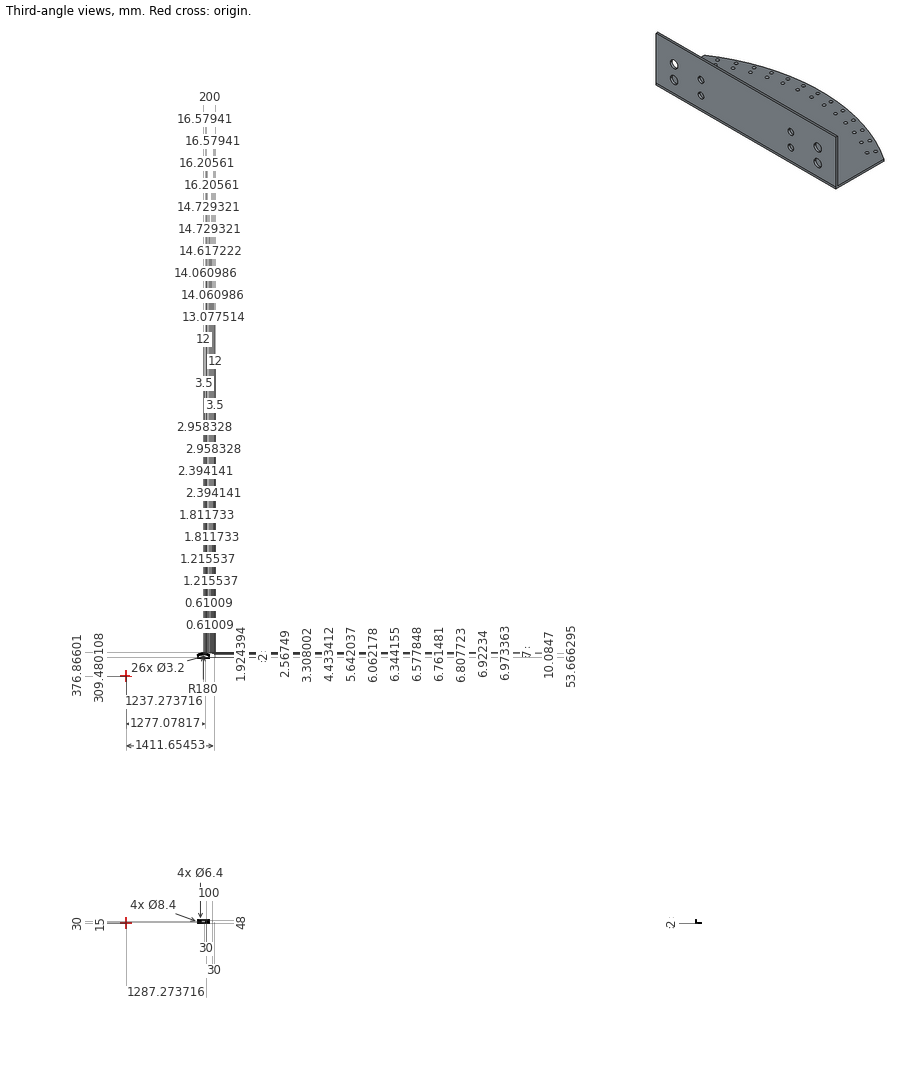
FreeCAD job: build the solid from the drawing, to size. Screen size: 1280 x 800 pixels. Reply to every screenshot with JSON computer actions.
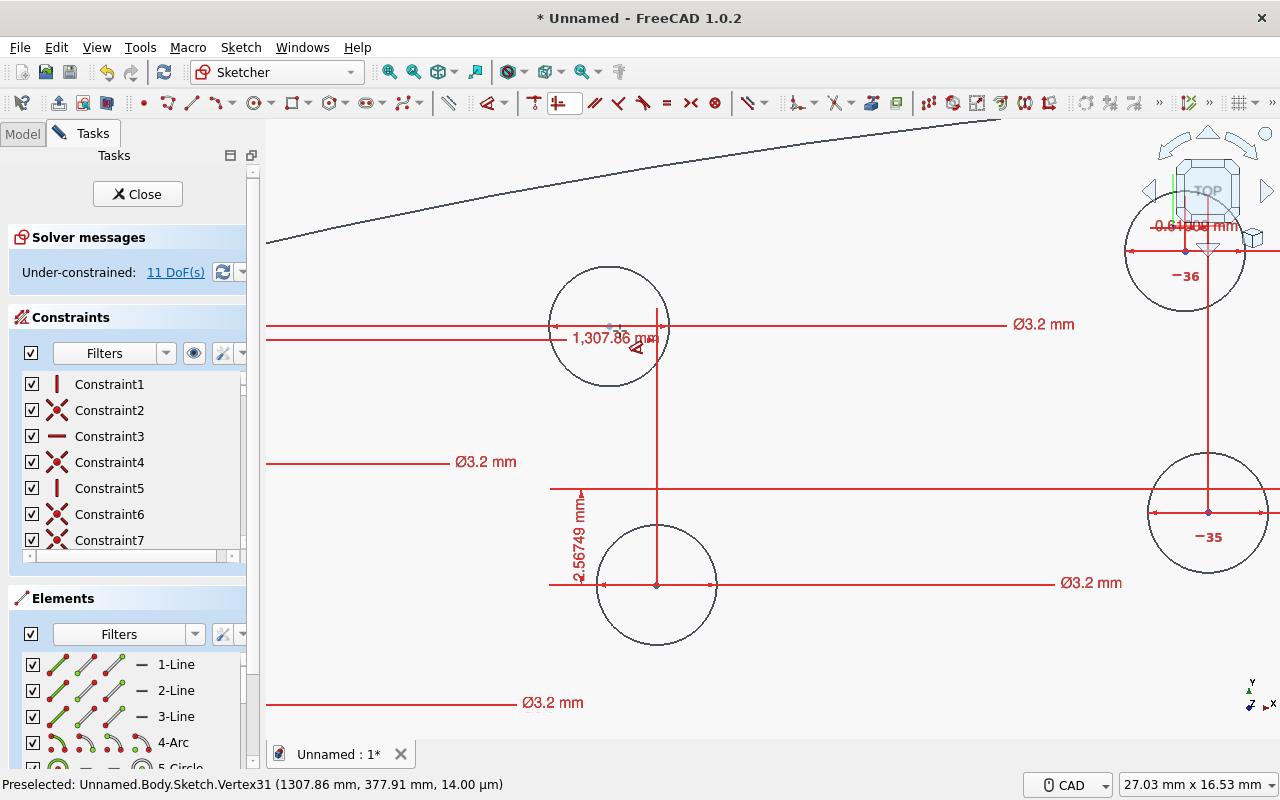
{"action": "left_click", "coordinate": [609, 326]}
{"action": "left_click", "coordinate": [633, 292]}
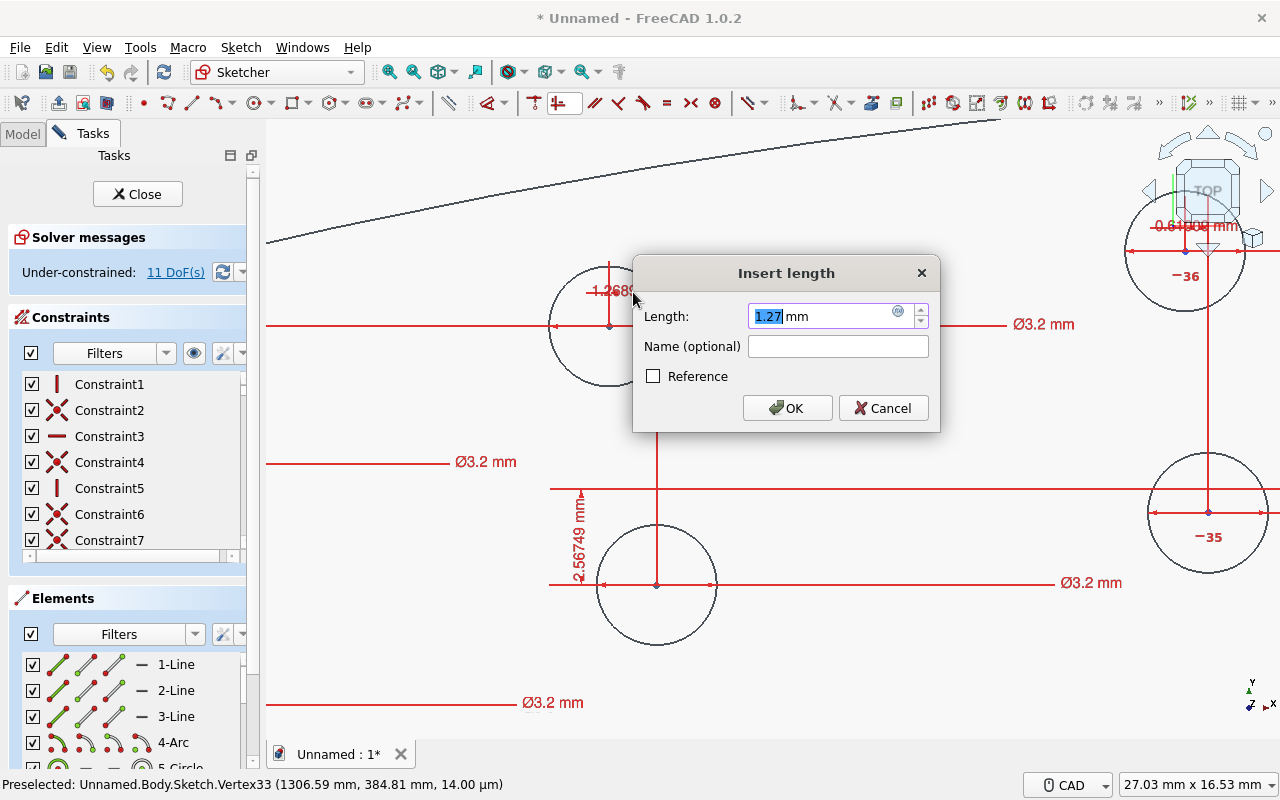
{"action": "type", "text": "1.215537"}
{"action": "key", "text": "Return"}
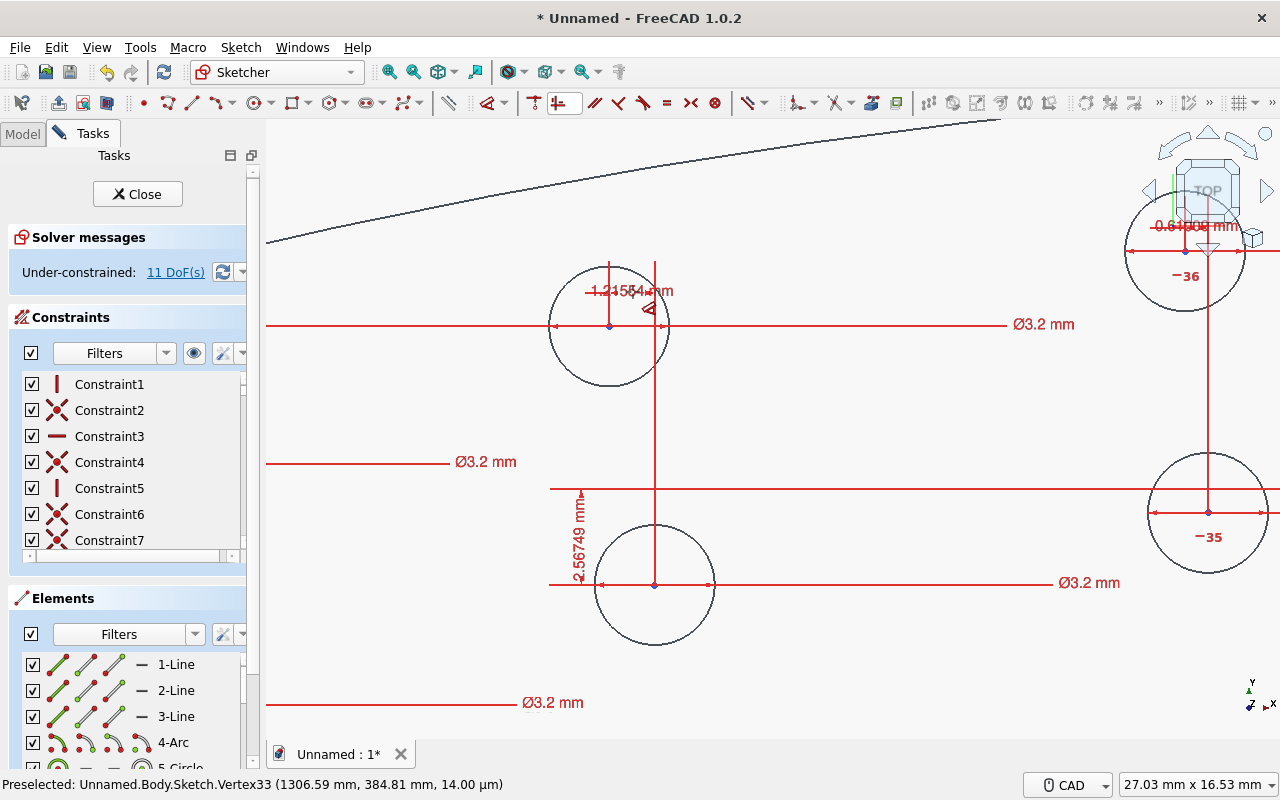
{"action": "scroll", "coordinate": [620, 331], "scroll_direction": "down", "scroll_amount": 13}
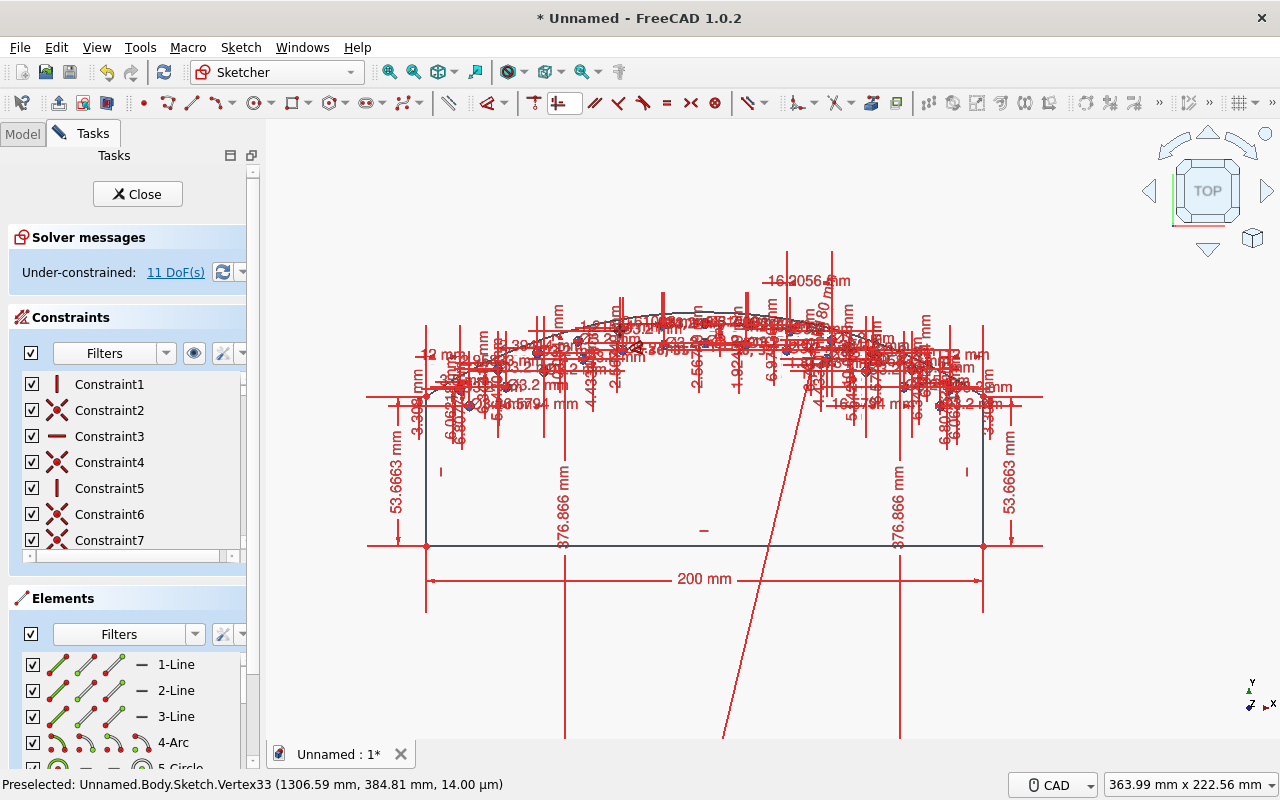
{"action": "scroll", "coordinate": [583, 359], "scroll_direction": "up", "scroll_amount": 11}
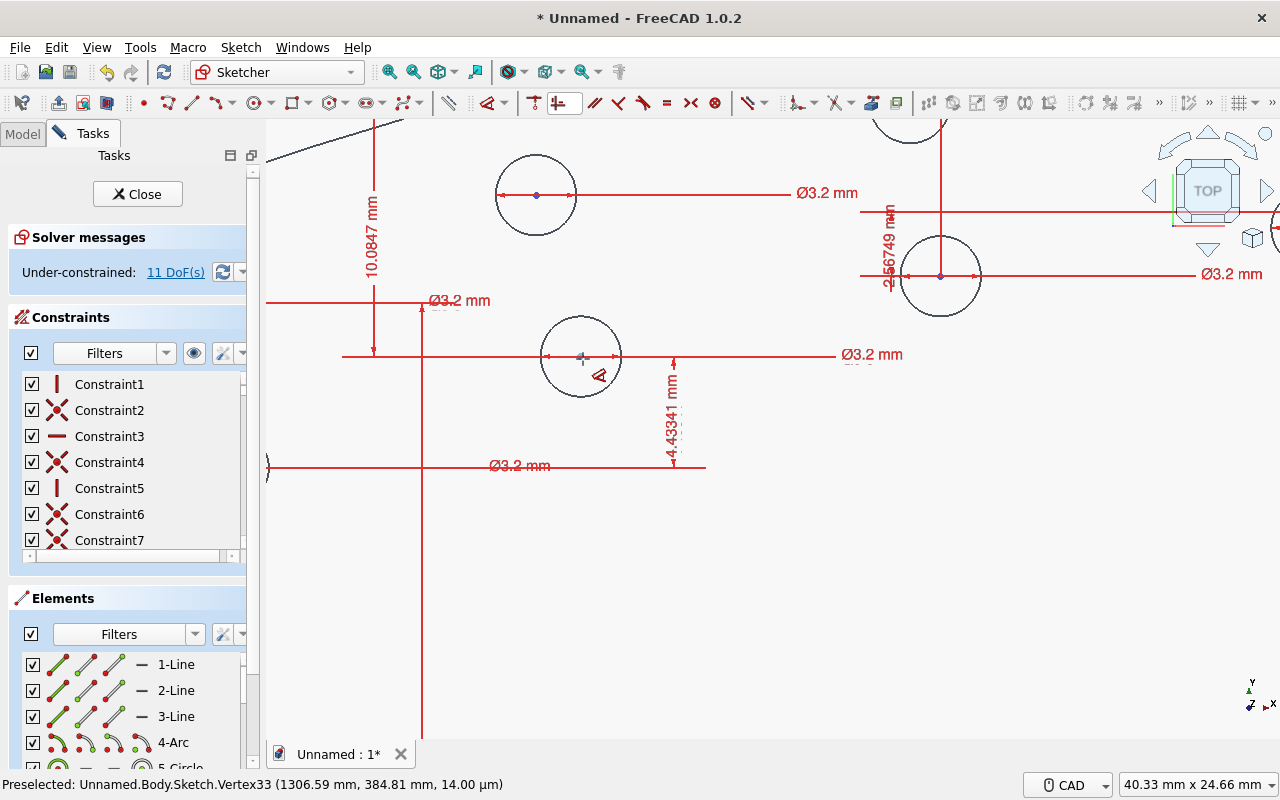
{"action": "left_click", "coordinate": [581, 357]}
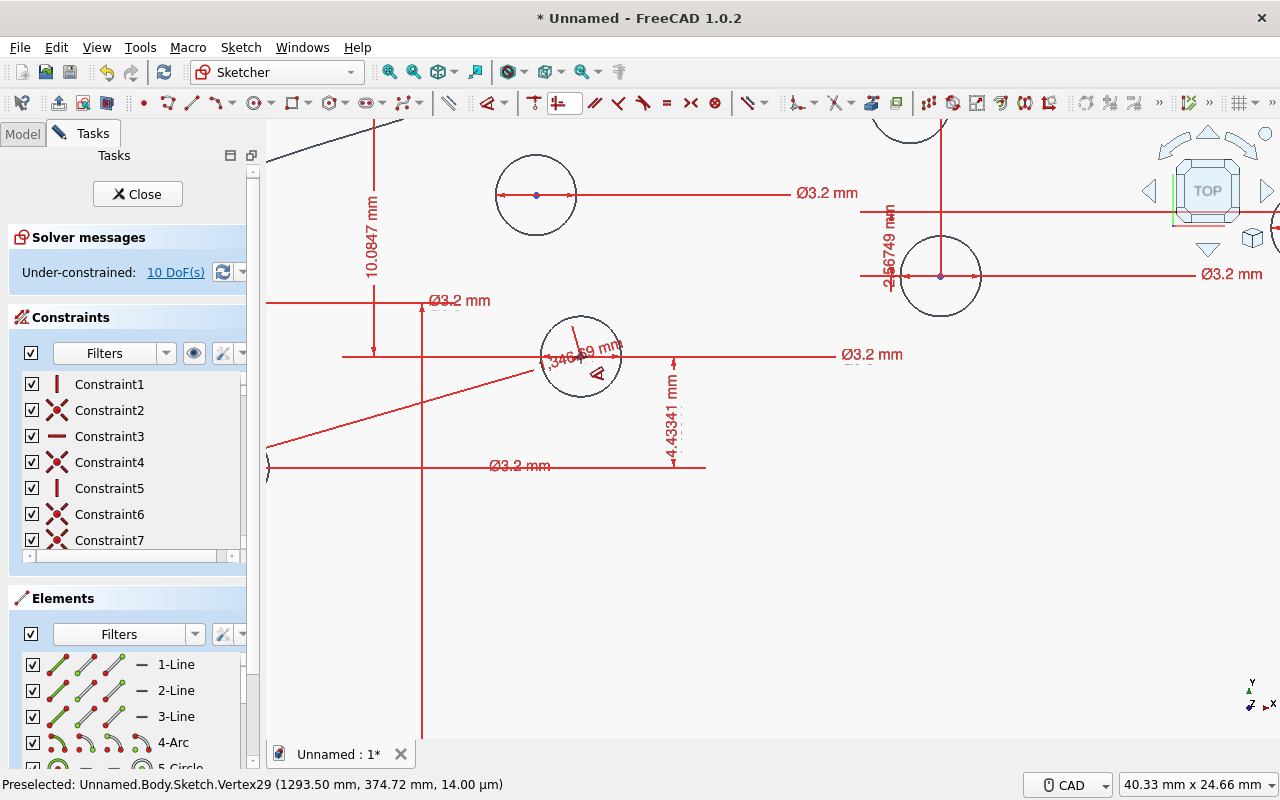
{"action": "left_click", "coordinate": [536, 195]}
{"action": "left_click", "coordinate": [559, 415]}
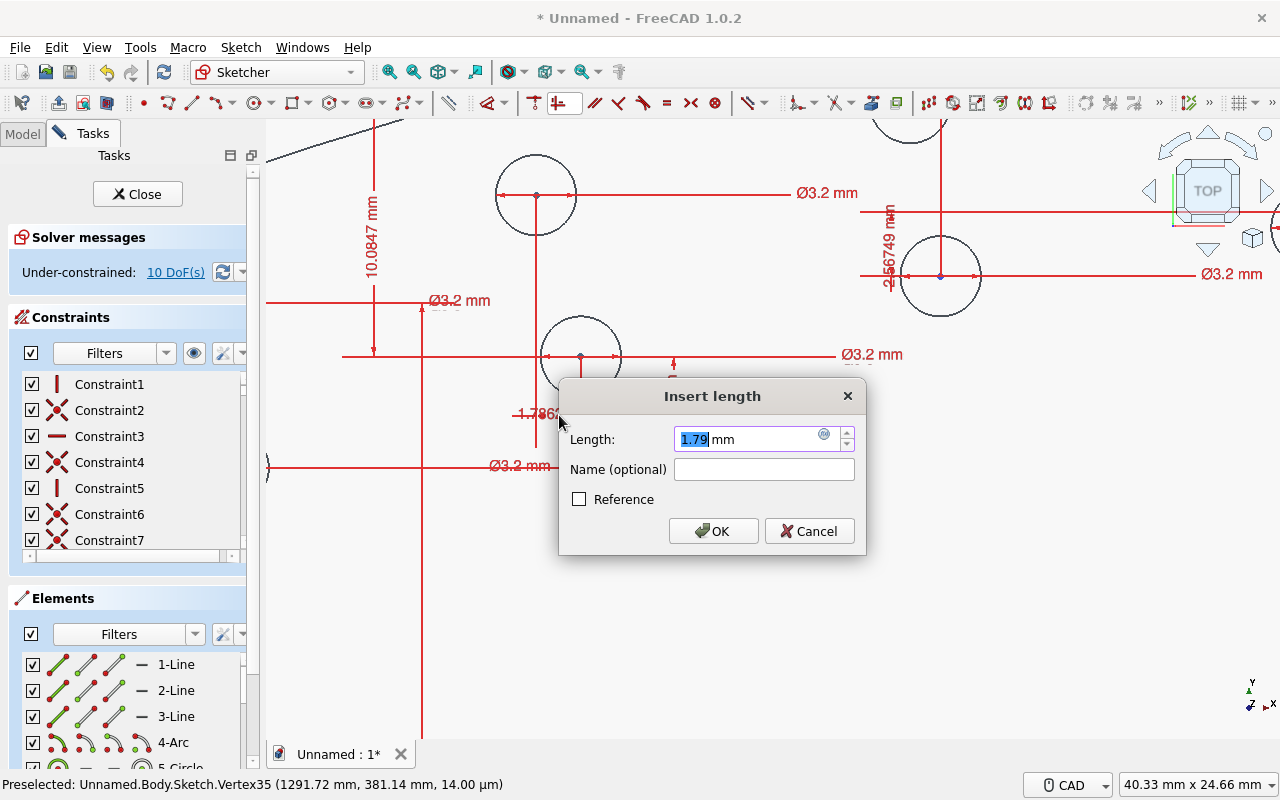
{"action": "type", "text": "1.811733"}
{"action": "key", "text": "Return"}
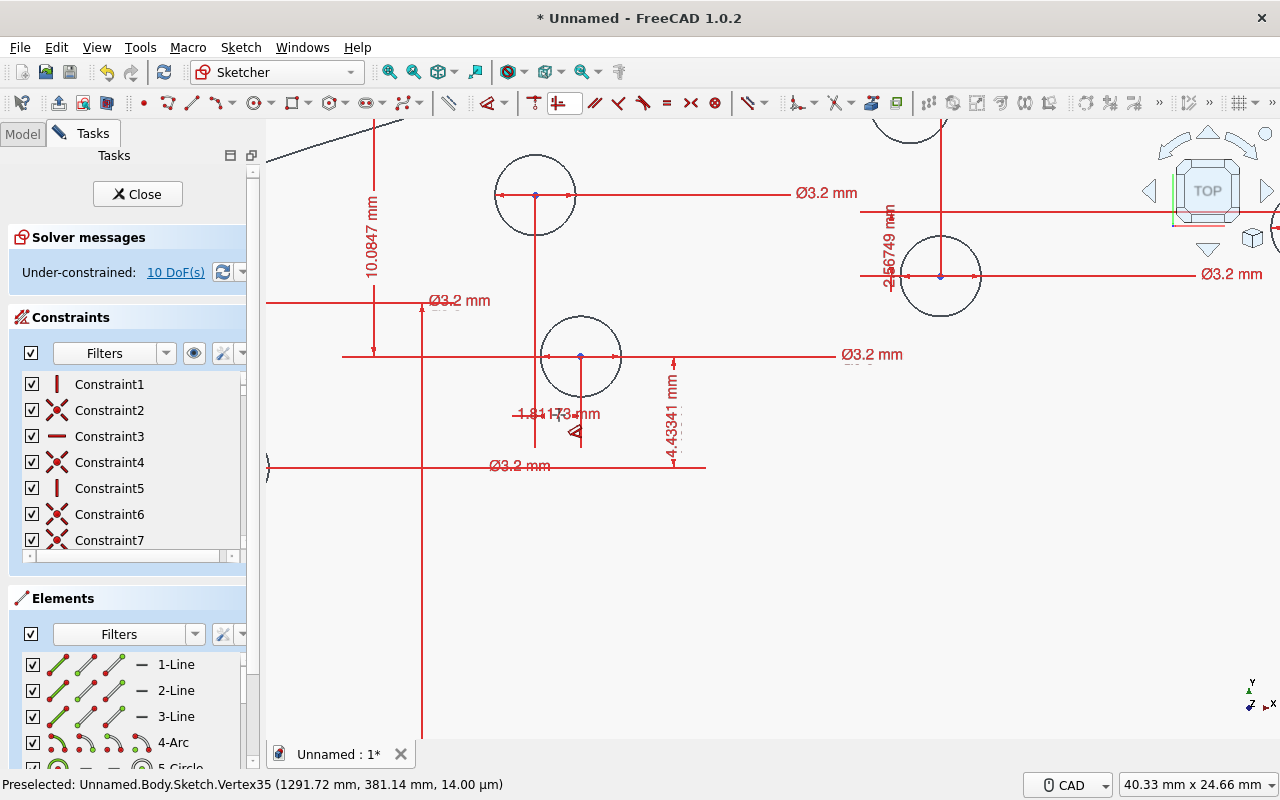
{"action": "scroll", "coordinate": [583, 359], "scroll_direction": "down", "scroll_amount": 11}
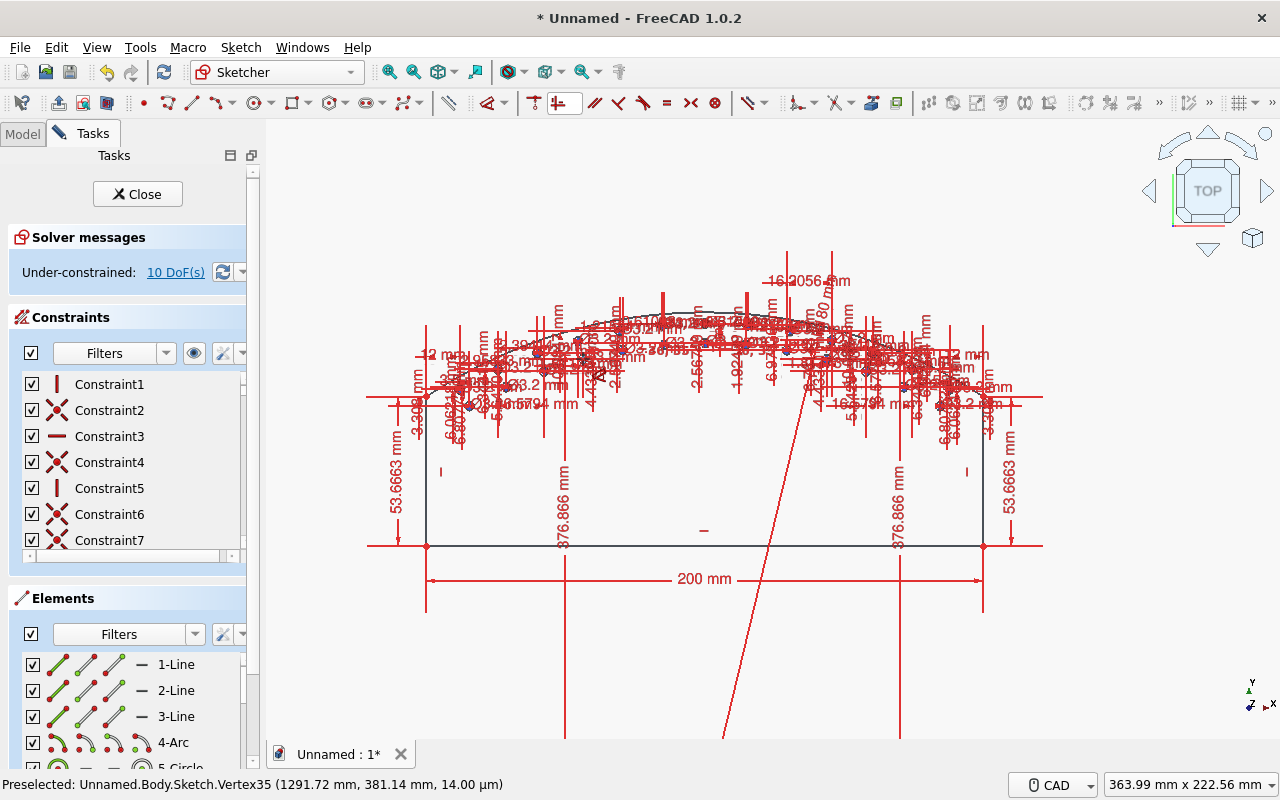
{"action": "left_click", "coordinate": [623, 350]}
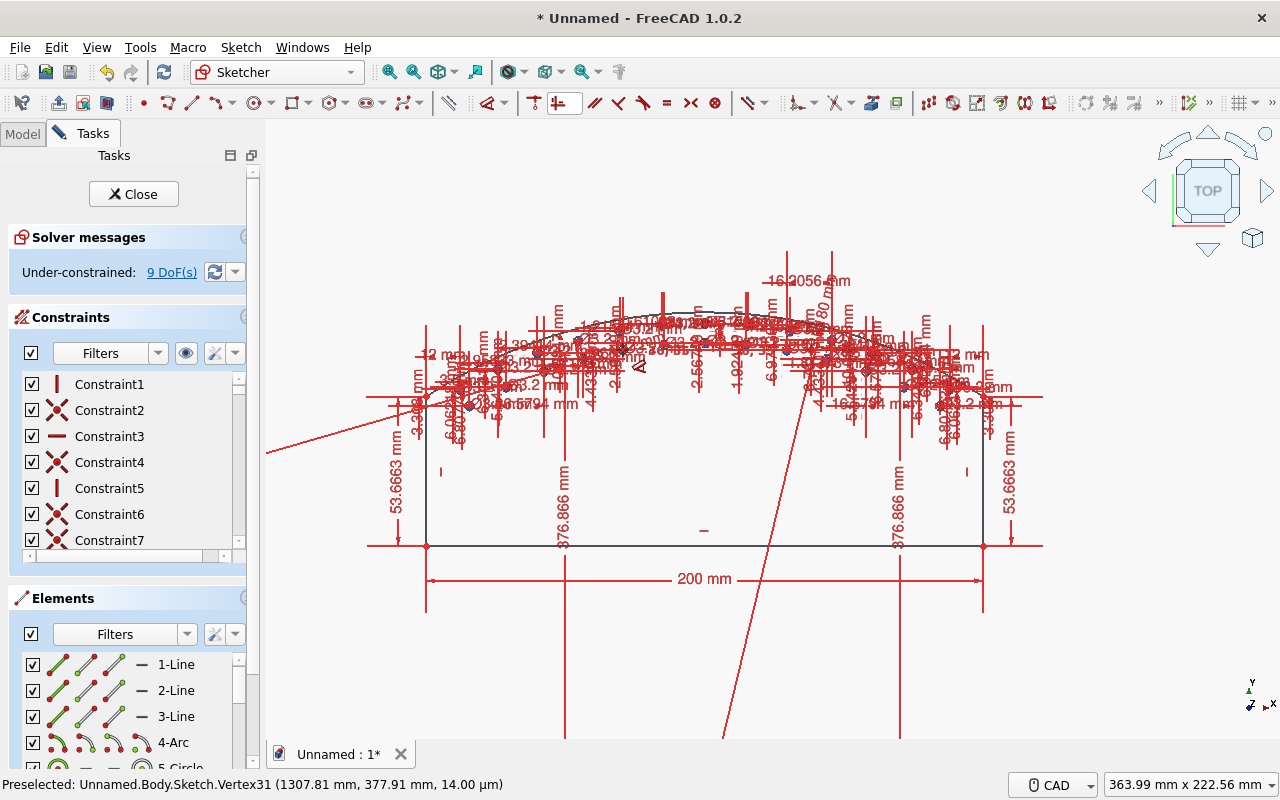
{"action": "left_click", "coordinate": [578, 341]}
{"action": "left_click", "coordinate": [590, 307]}